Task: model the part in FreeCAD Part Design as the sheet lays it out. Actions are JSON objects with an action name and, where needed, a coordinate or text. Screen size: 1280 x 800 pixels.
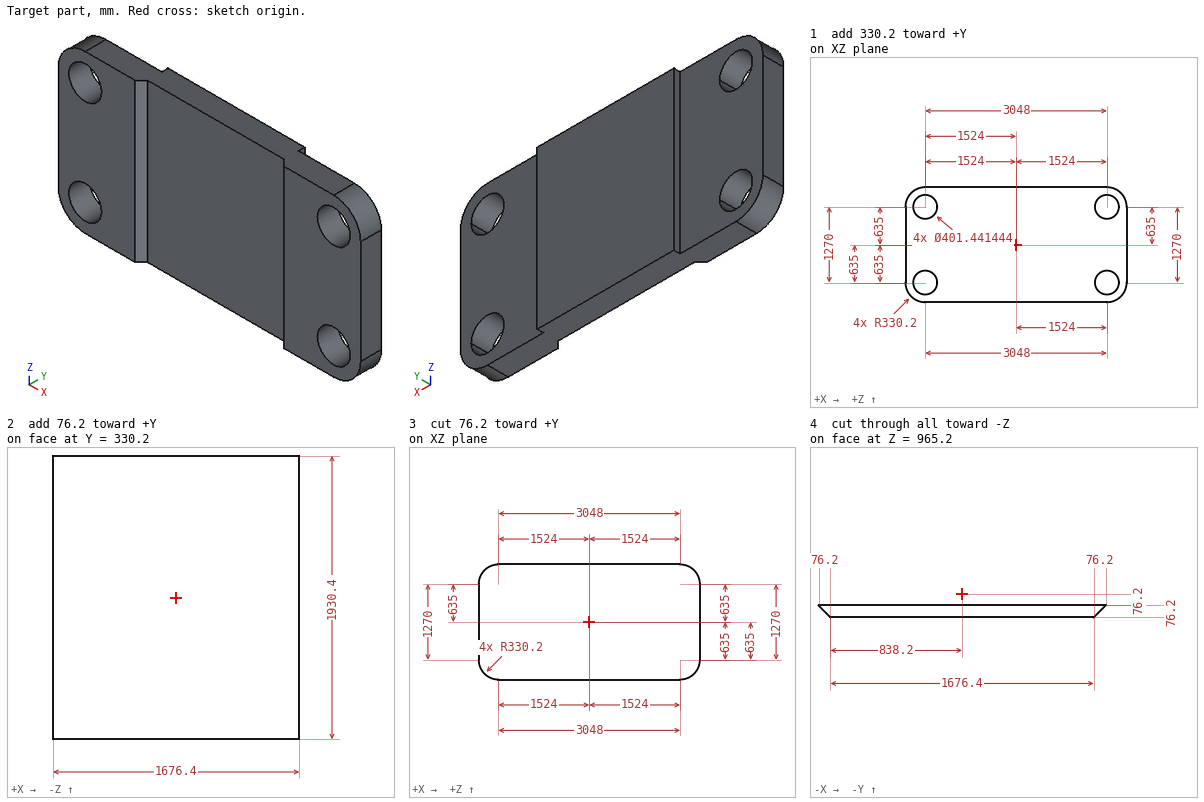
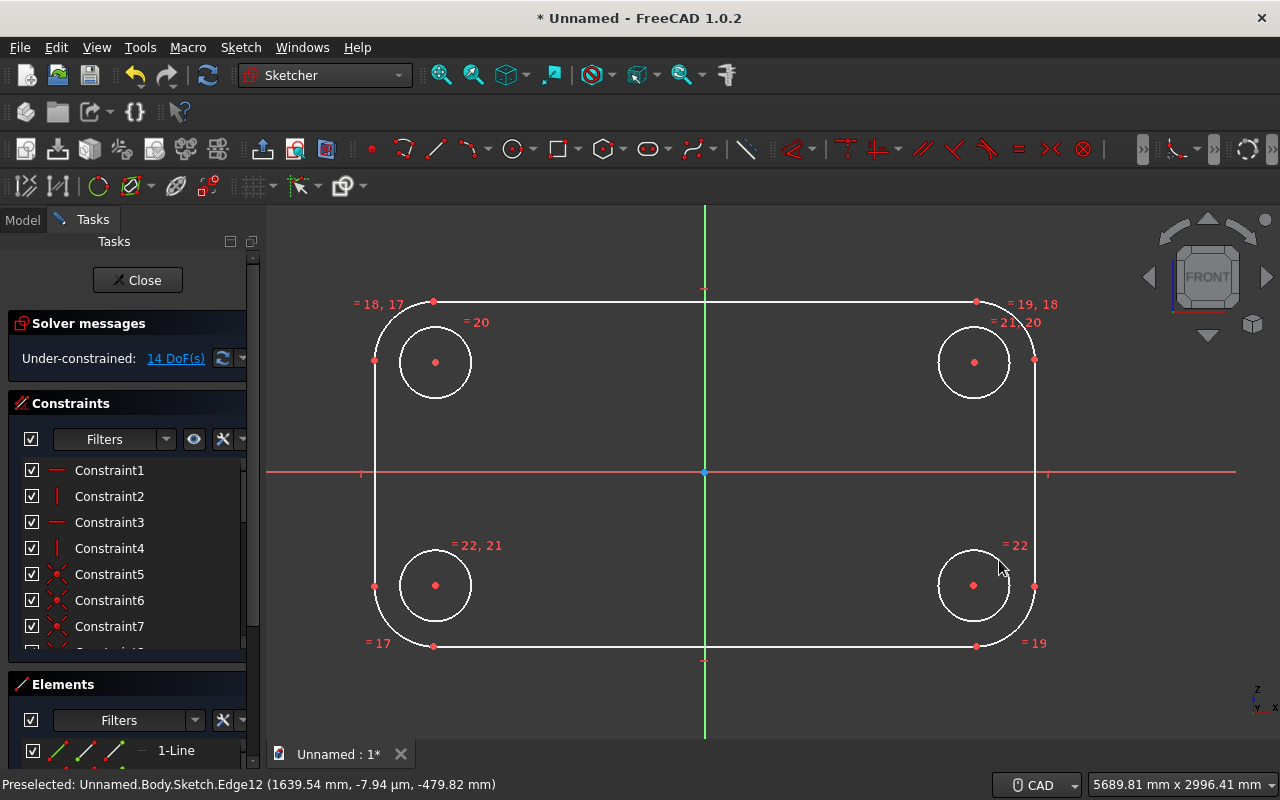
{"action": "left_click", "coordinate": [381, 614]}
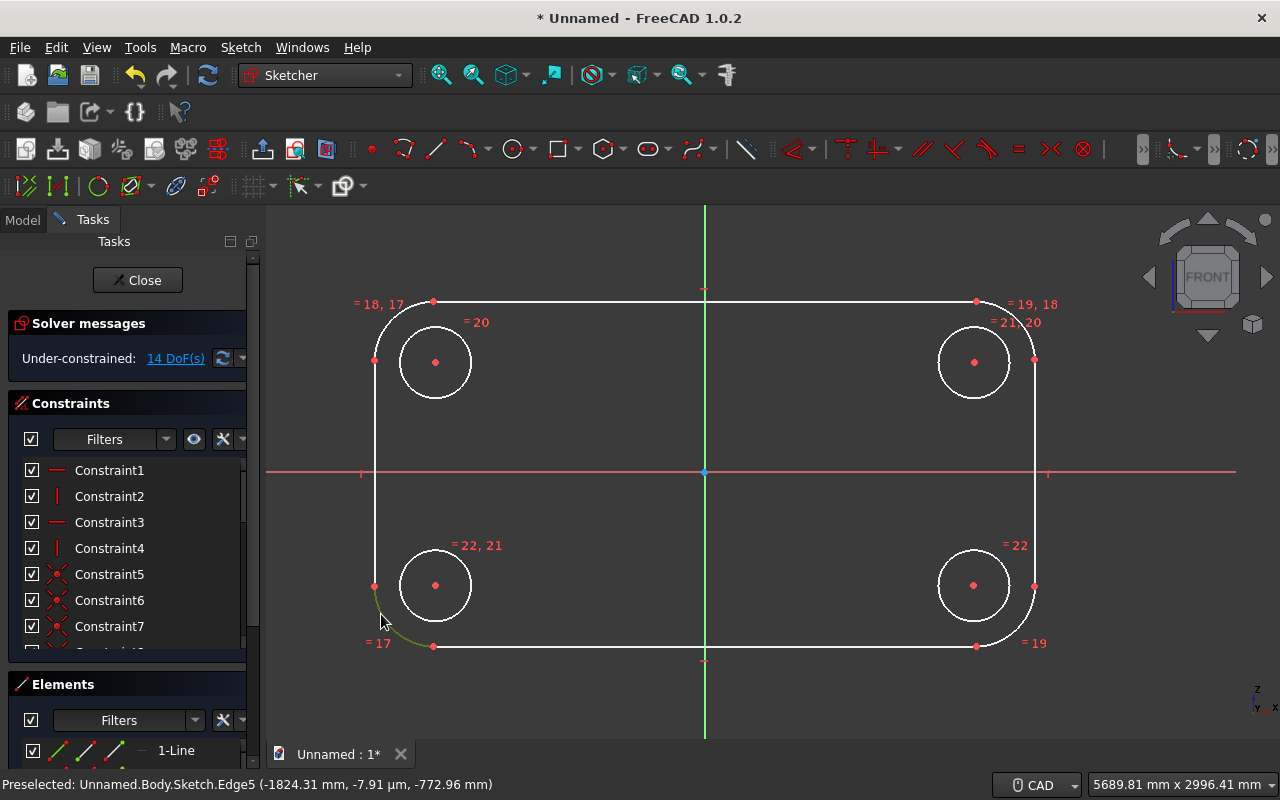
{"action": "left_click", "coordinate": [814, 150]}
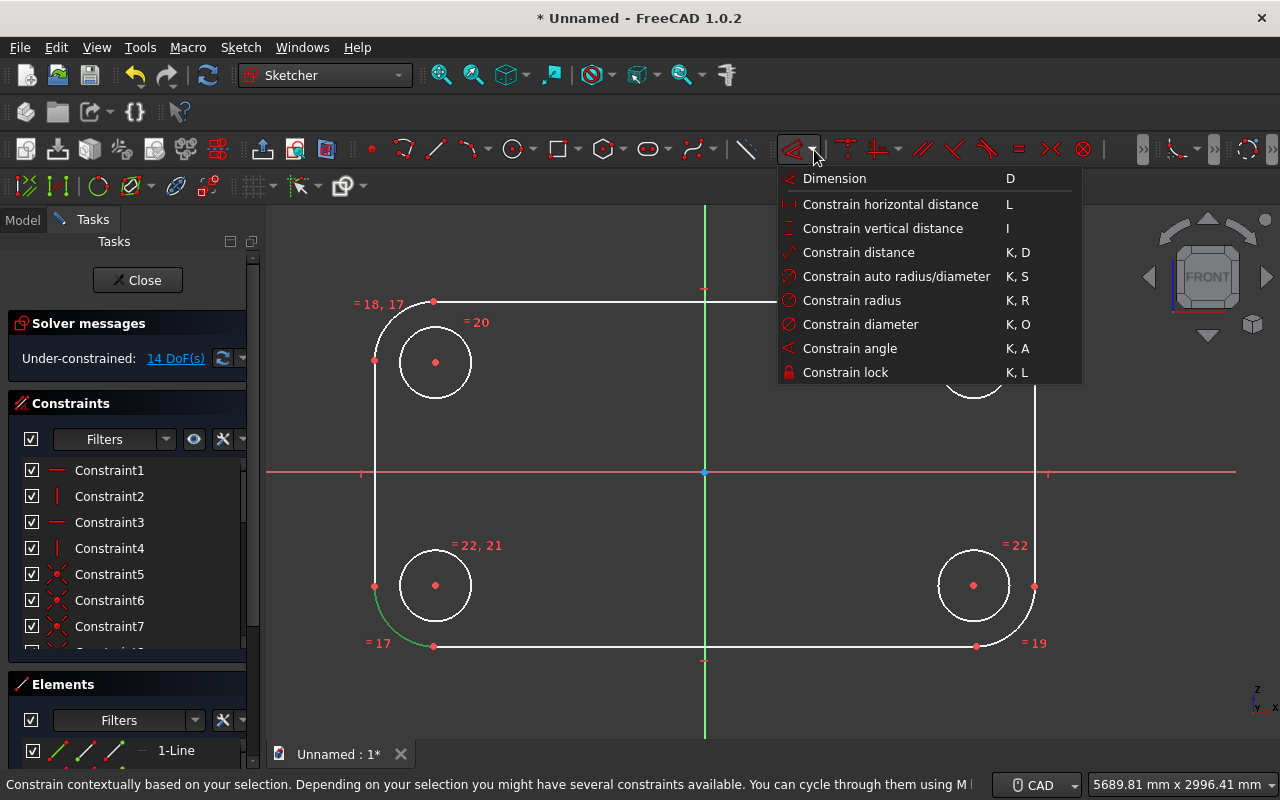
{"action": "left_click", "coordinate": [930, 300]}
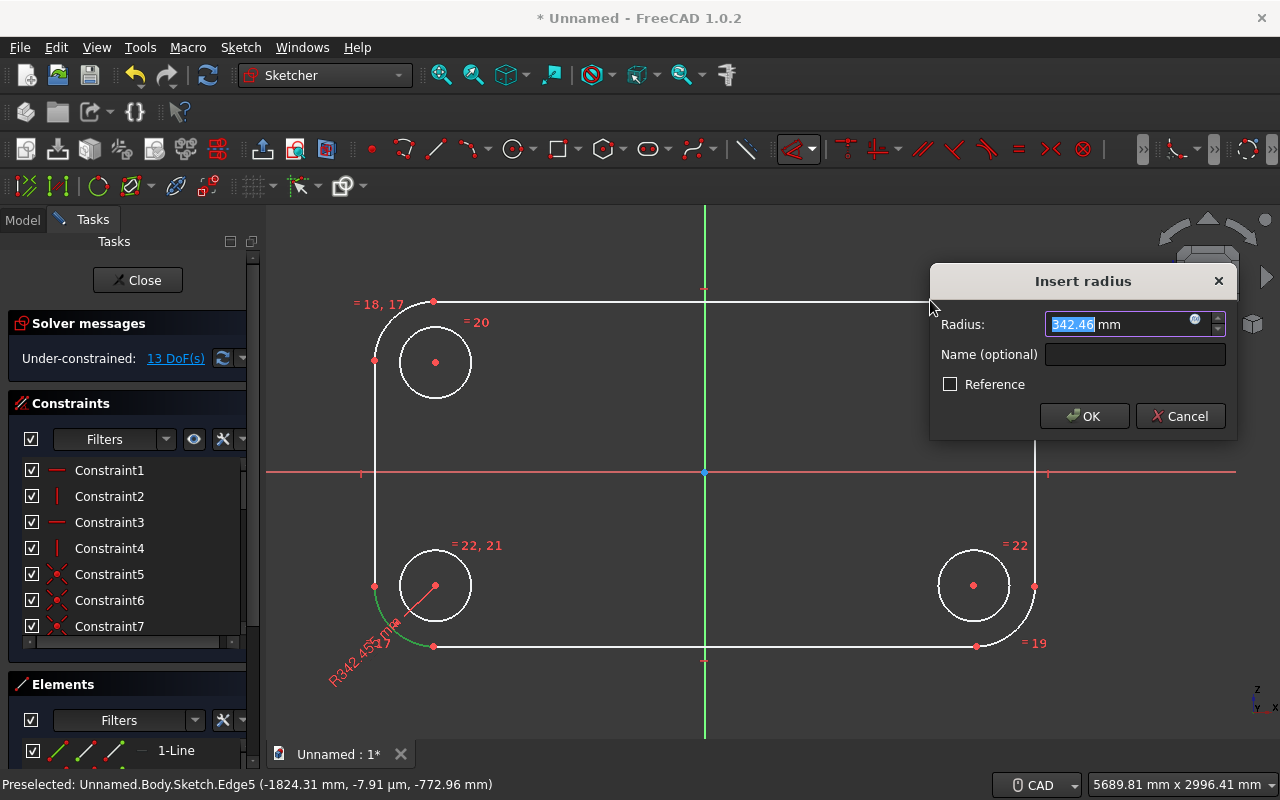
{"action": "type", "text": "330.2"}
{"action": "key", "text": "Return"}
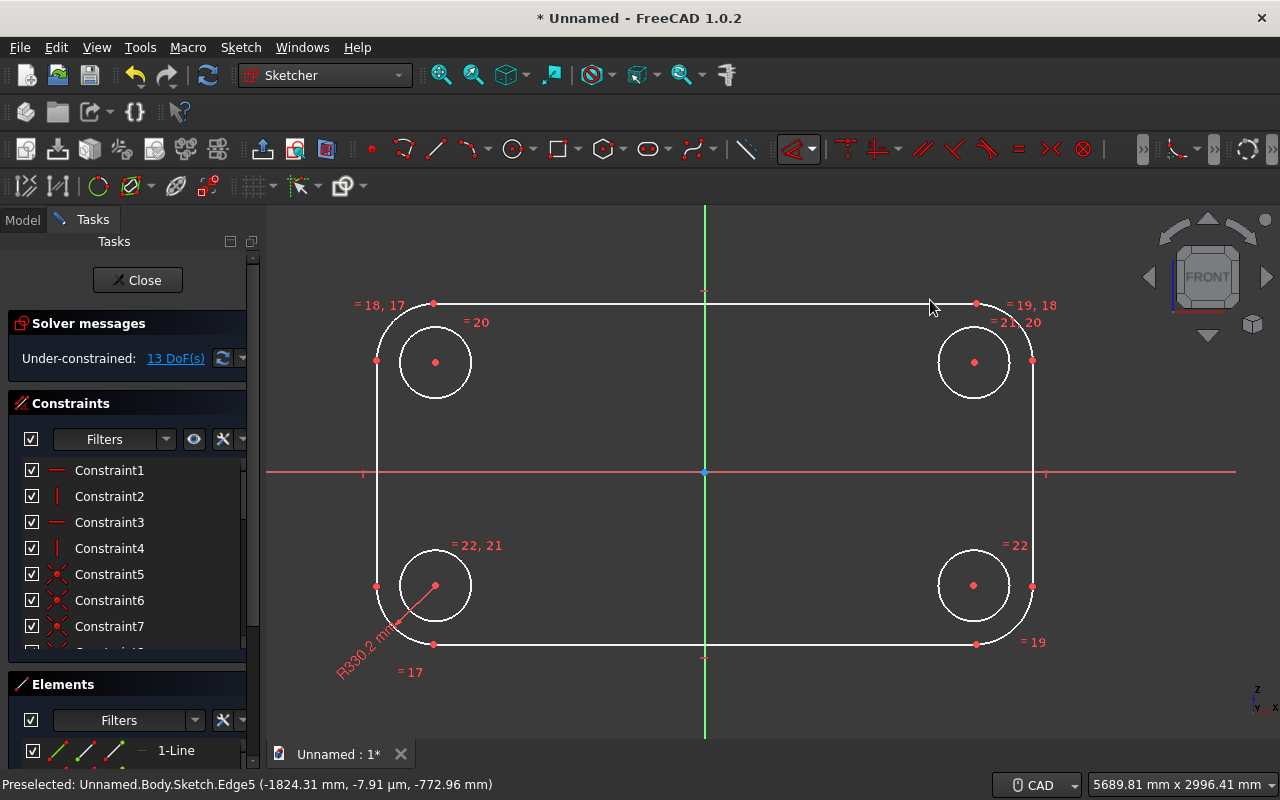
{"action": "left_click", "coordinate": [461, 337]}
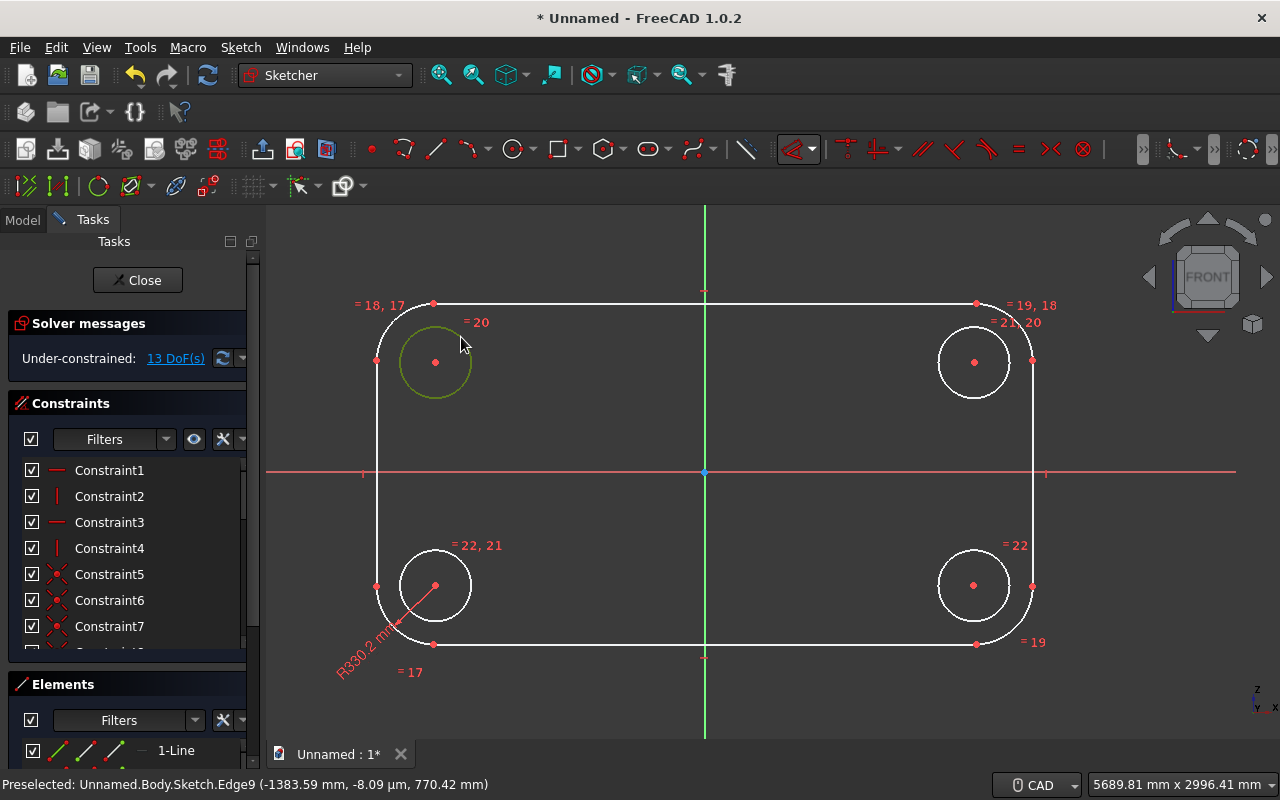
{"action": "key", "text": "k o"}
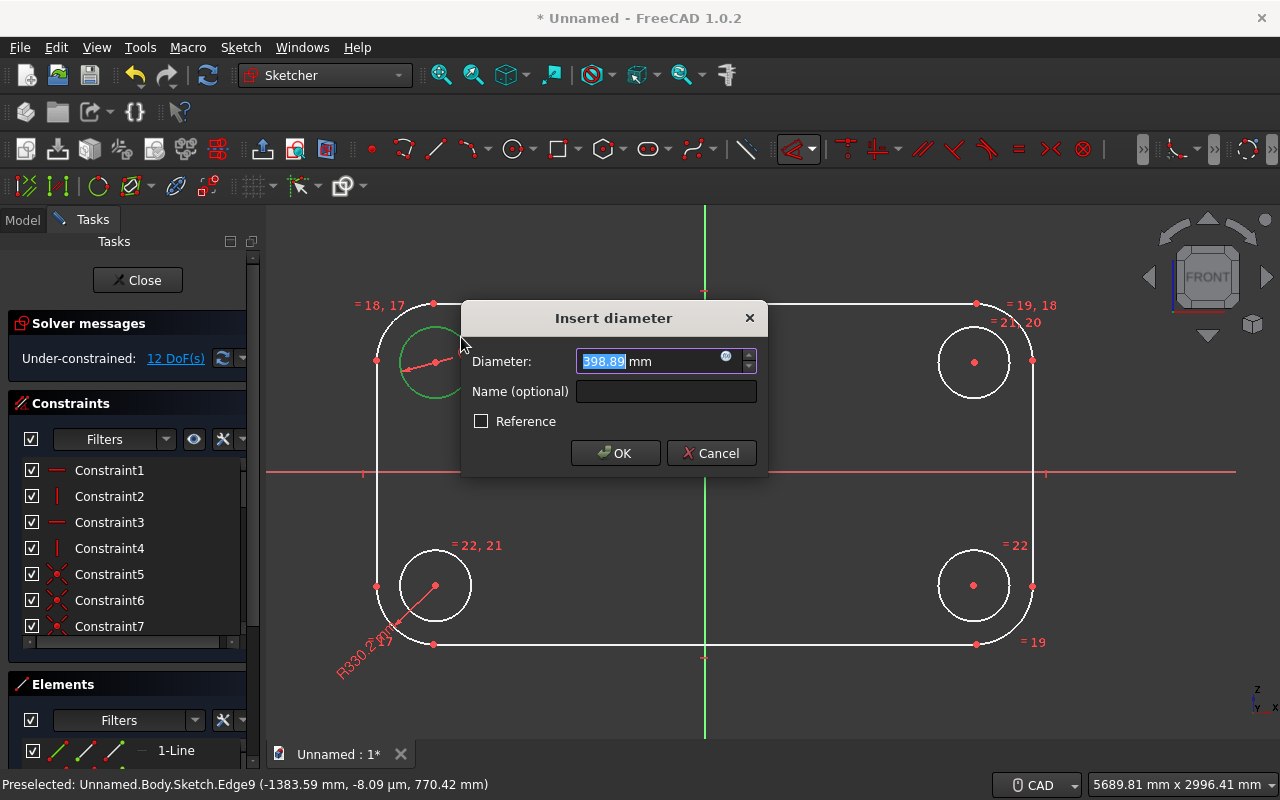
{"action": "type", "text": "401.441444"}
{"action": "key", "text": "Return"}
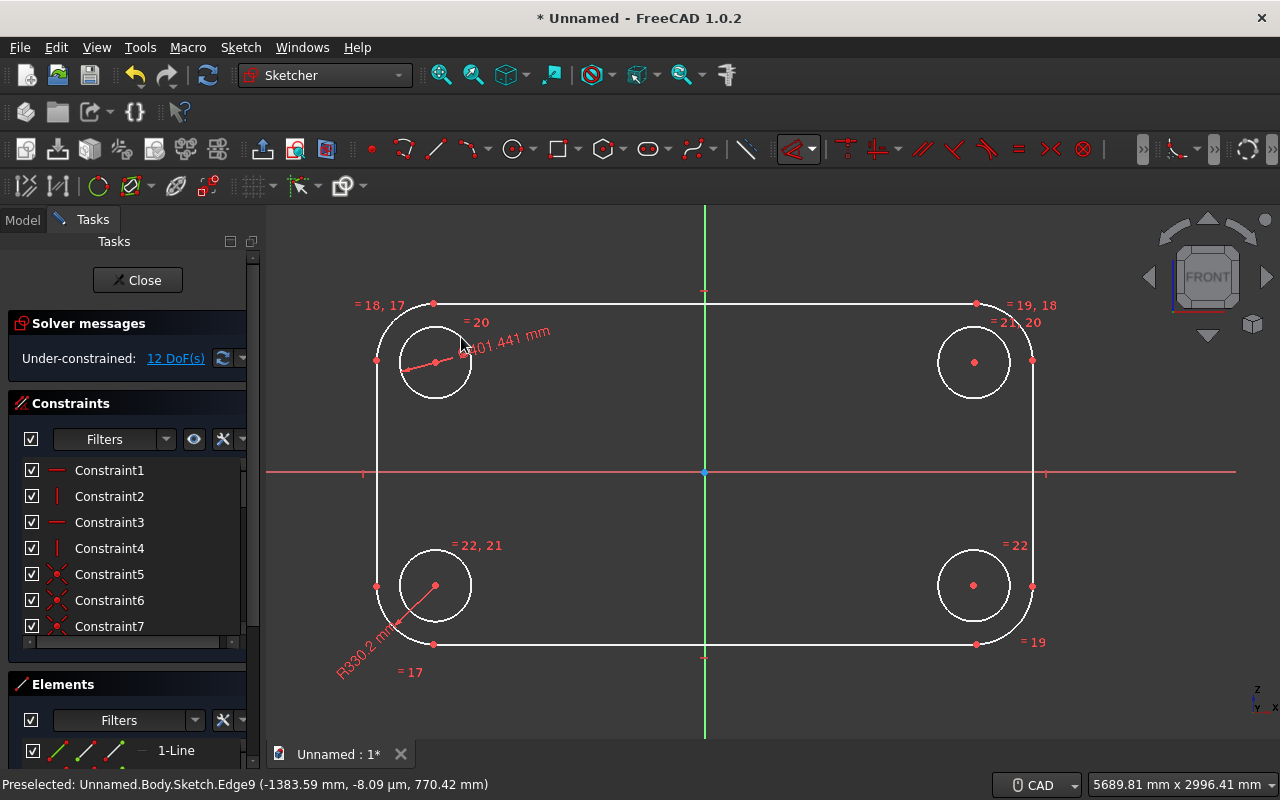
{"action": "left_click", "coordinate": [436, 363]}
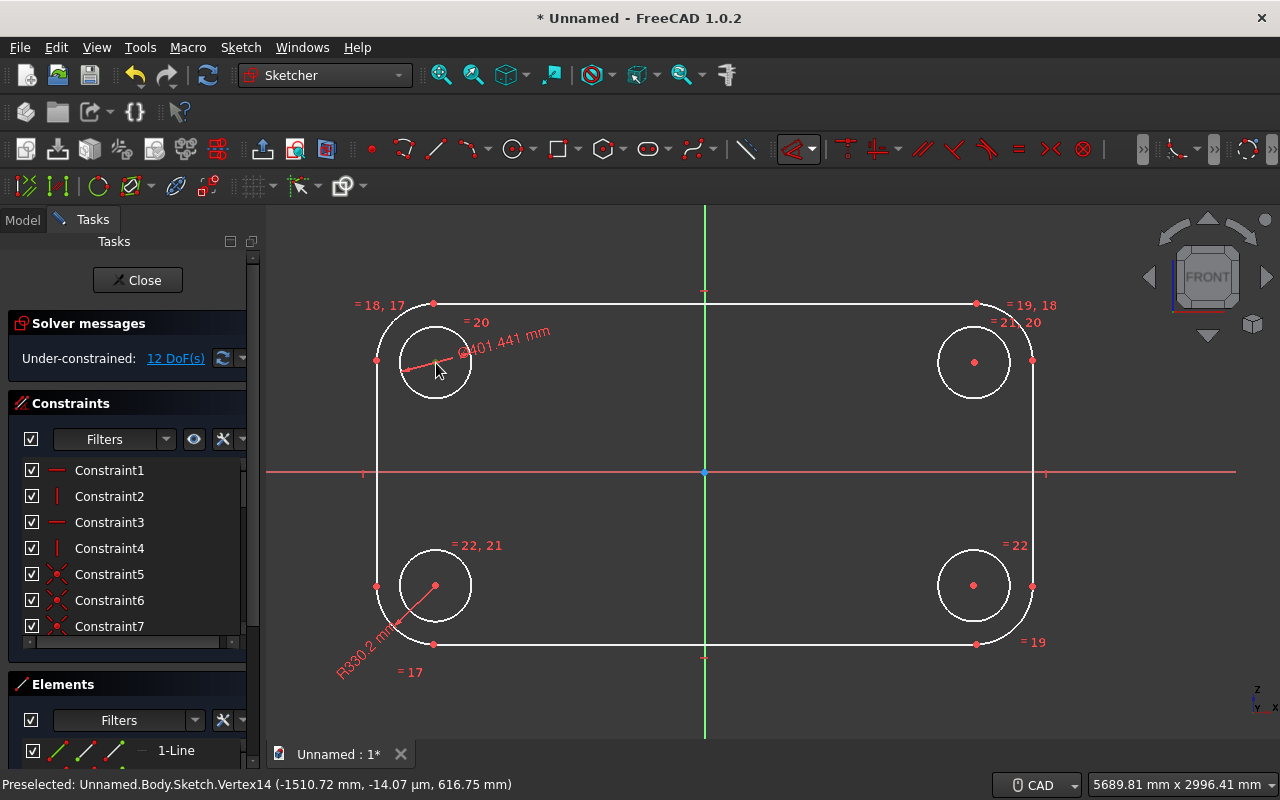
{"action": "left_click", "coordinate": [814, 150]}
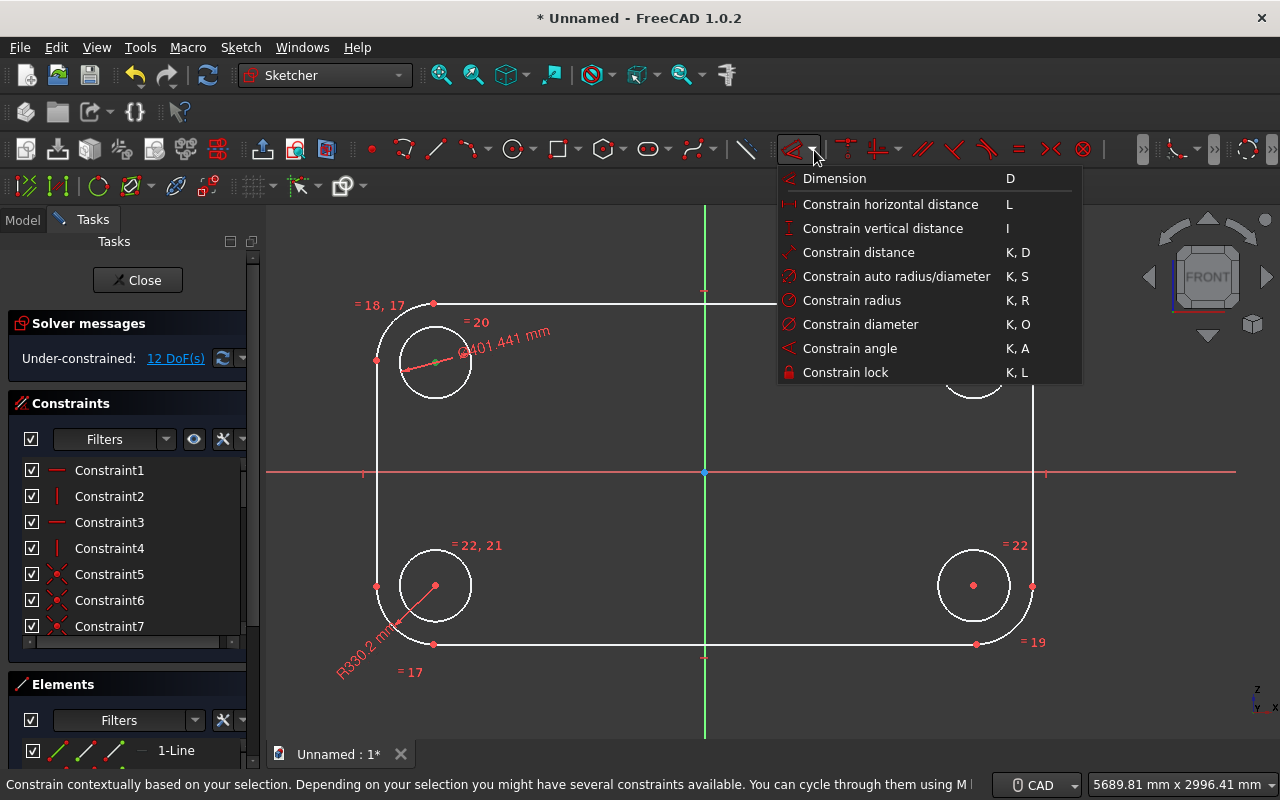
{"action": "left_click", "coordinate": [930, 228]}